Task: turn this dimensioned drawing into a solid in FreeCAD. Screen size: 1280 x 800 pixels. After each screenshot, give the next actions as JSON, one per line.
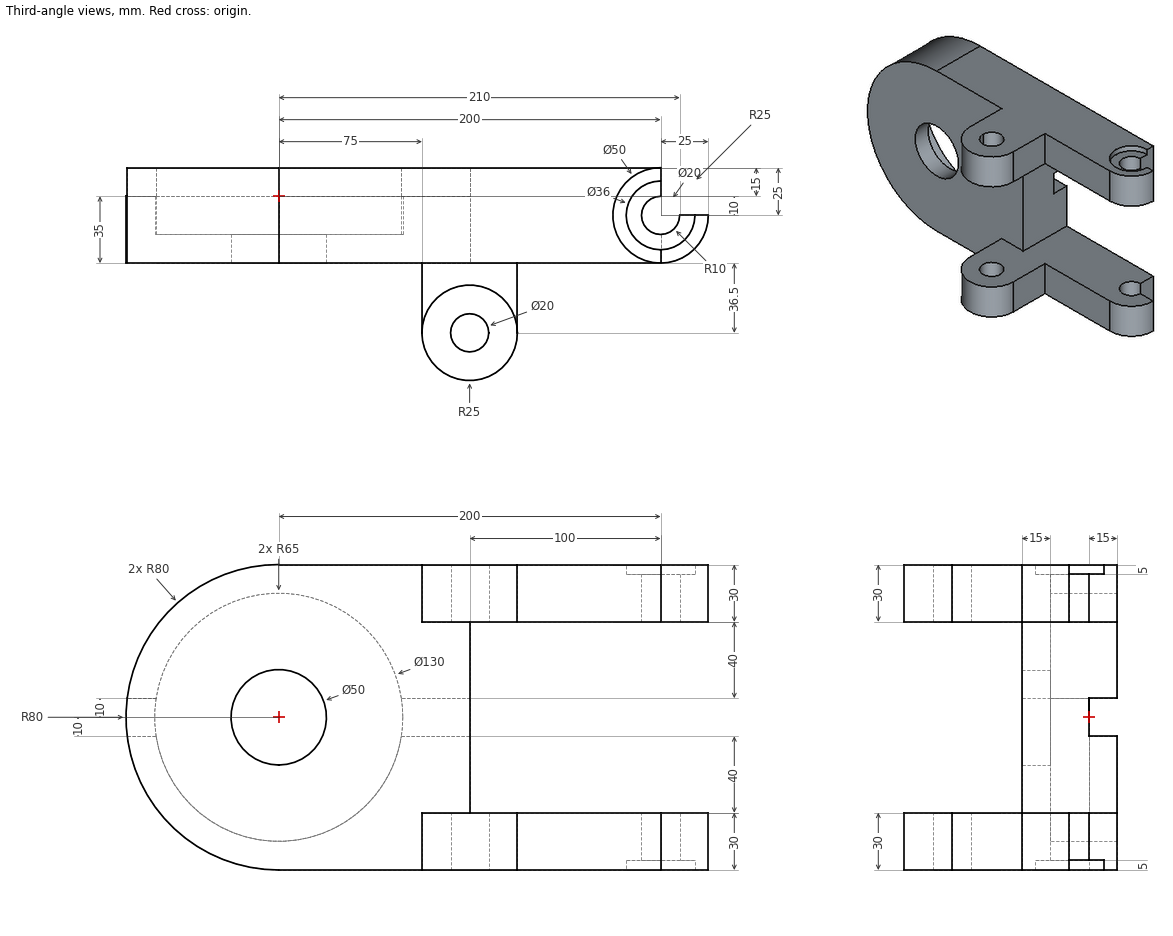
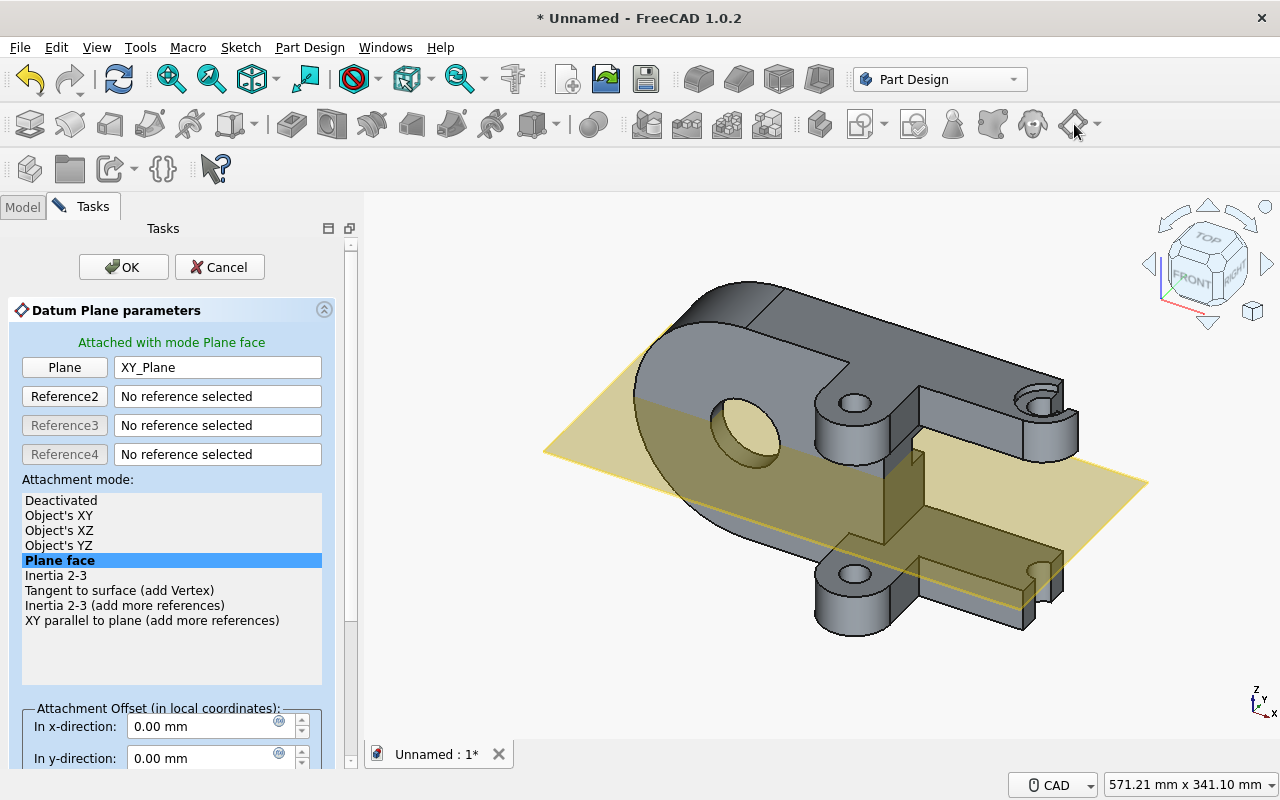
{"action": "scroll", "coordinate": [351, 503], "scroll_direction": "down", "scroll_amount": 2}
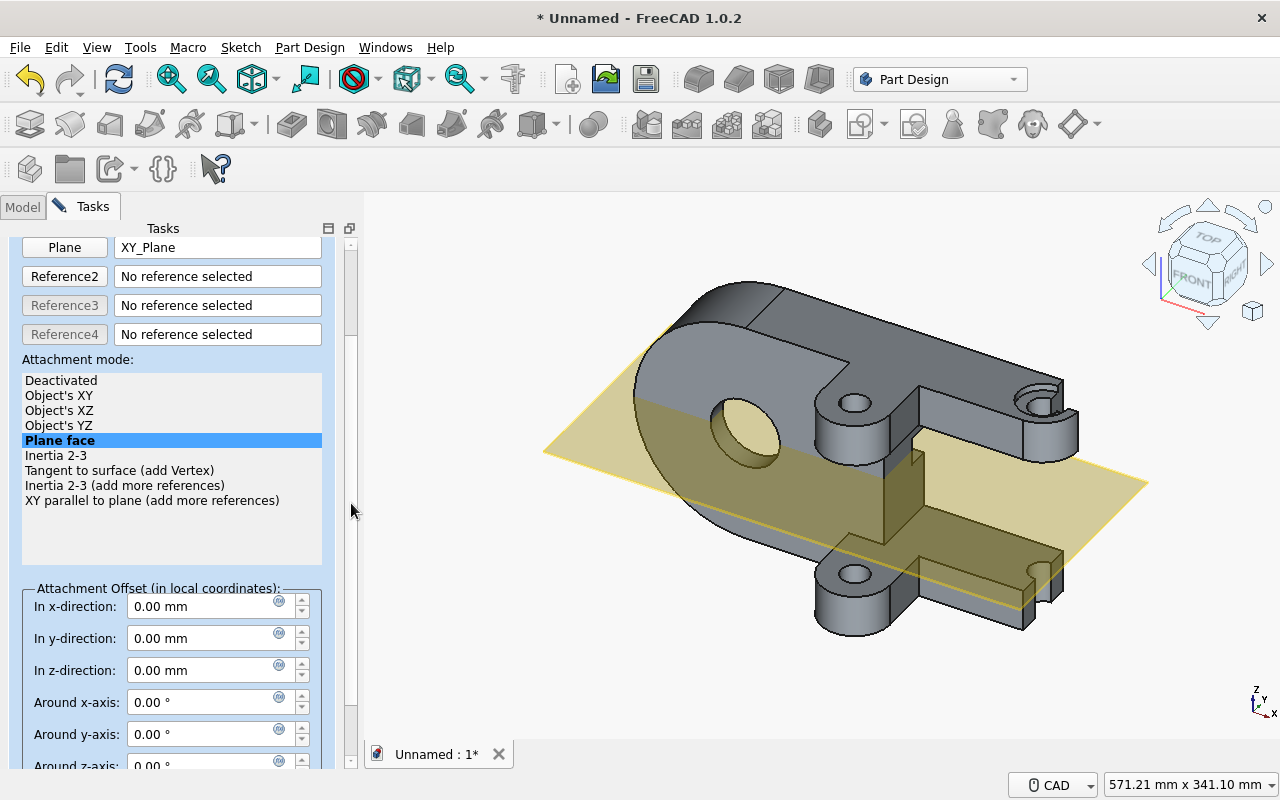
{"action": "triple_click", "coordinate": [210, 670]}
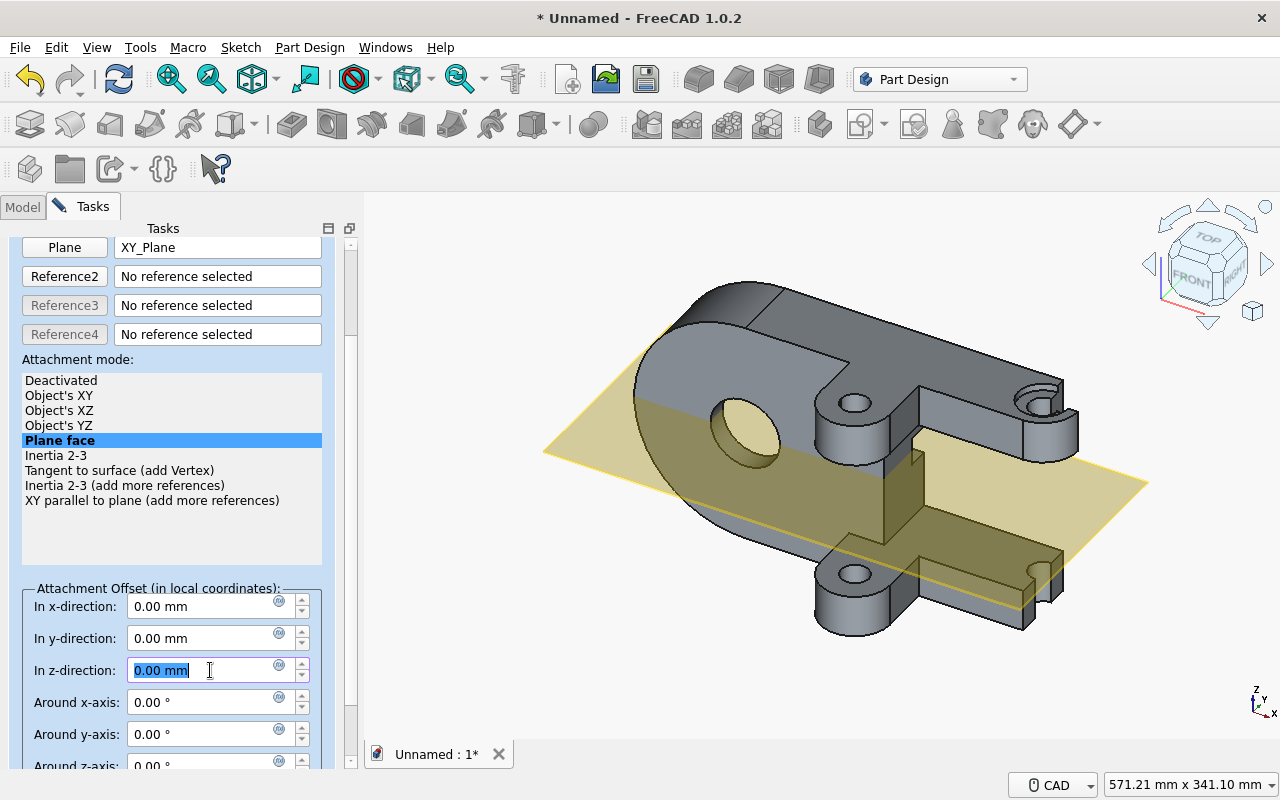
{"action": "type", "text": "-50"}
{"action": "key", "text": "Tab"}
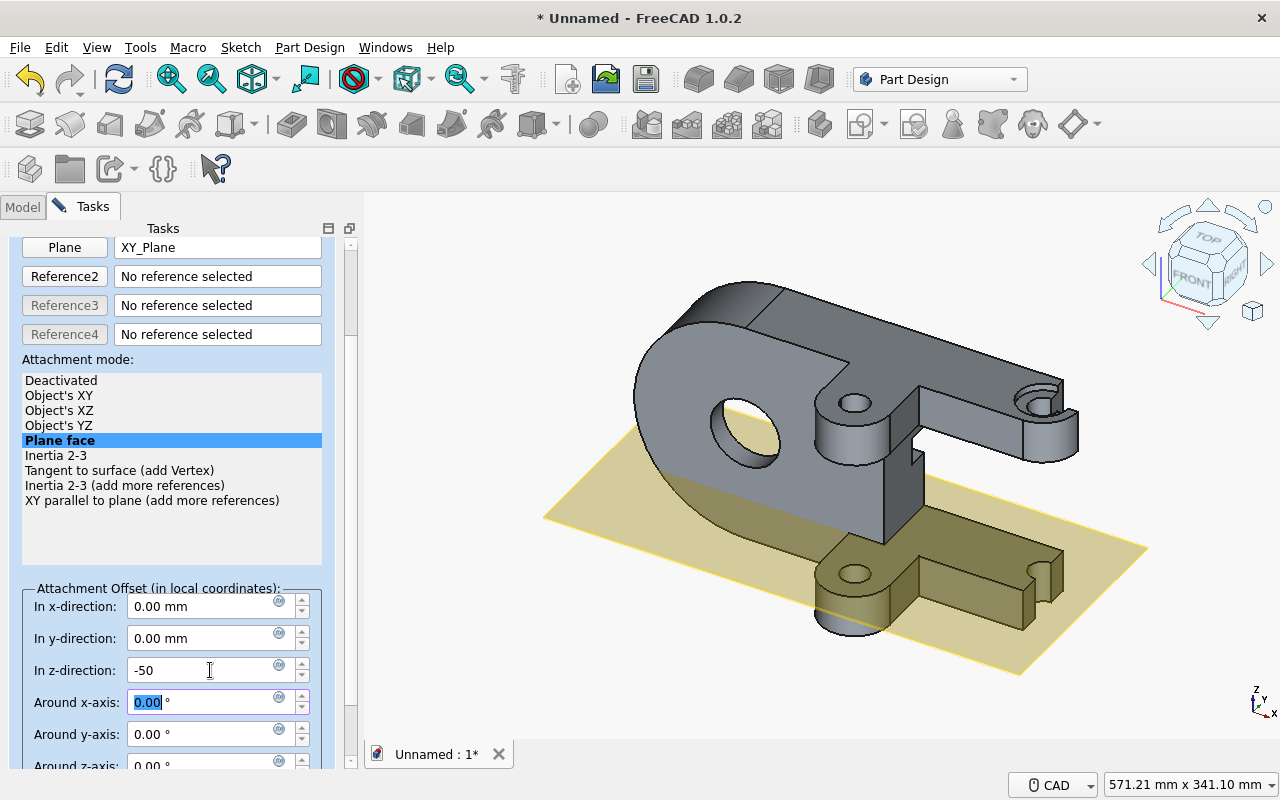
{"action": "scroll", "coordinate": [351, 503], "scroll_direction": "up", "scroll_amount": 3}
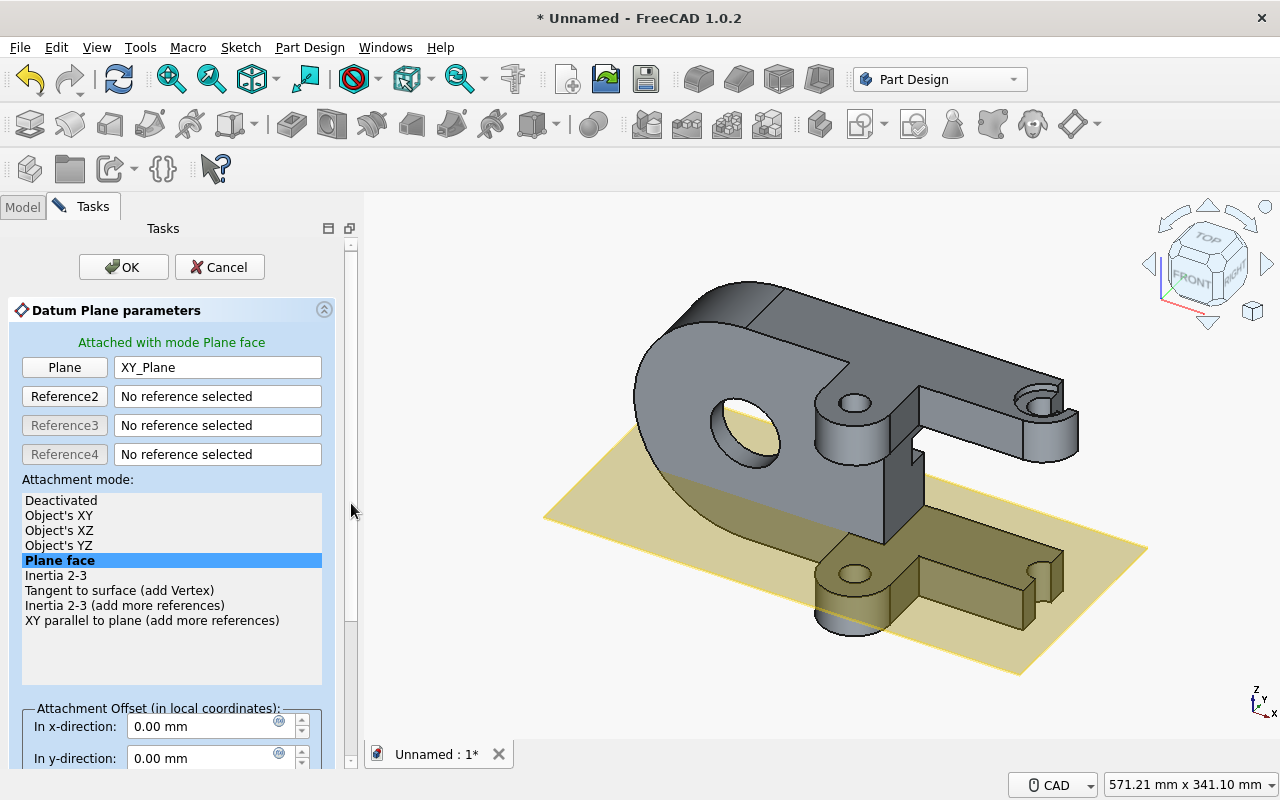
{"action": "left_click", "coordinate": [124, 267]}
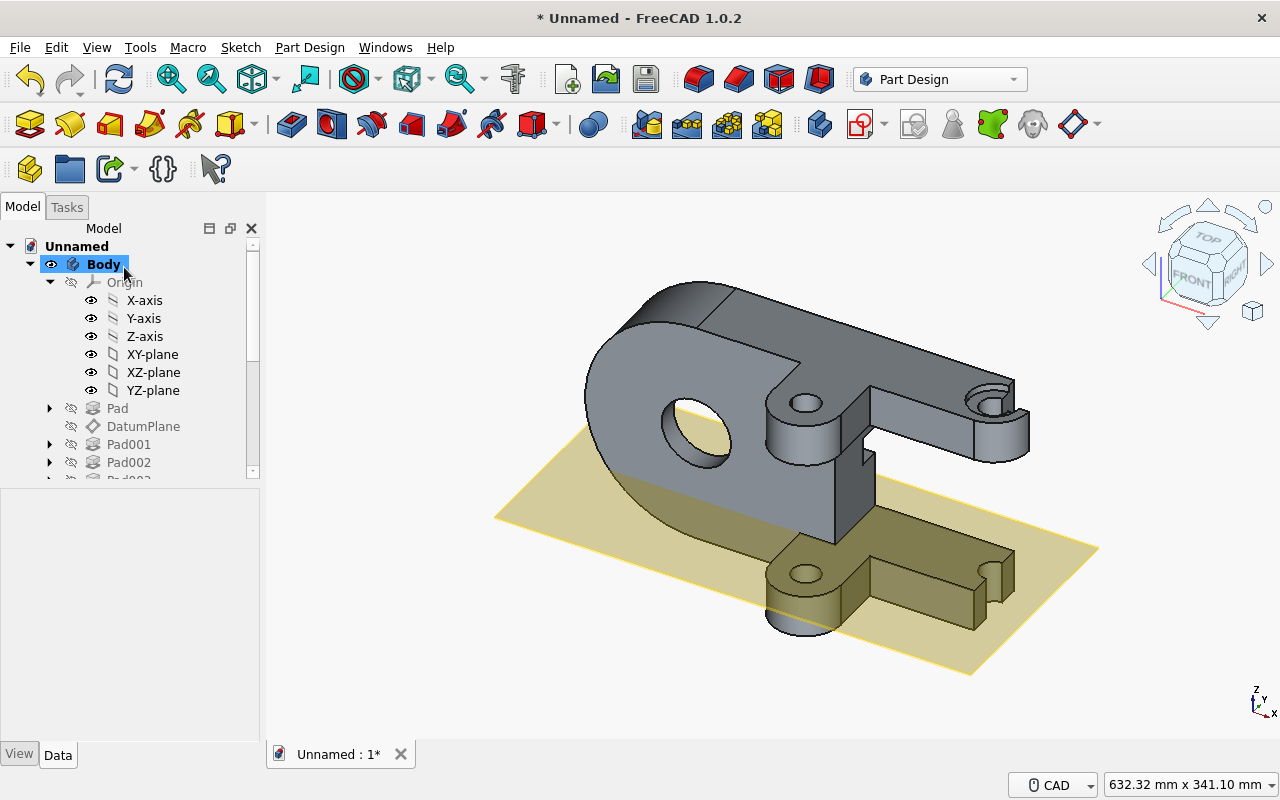
{"action": "scroll", "coordinate": [100, 350], "scroll_direction": "down", "scroll_amount": 3}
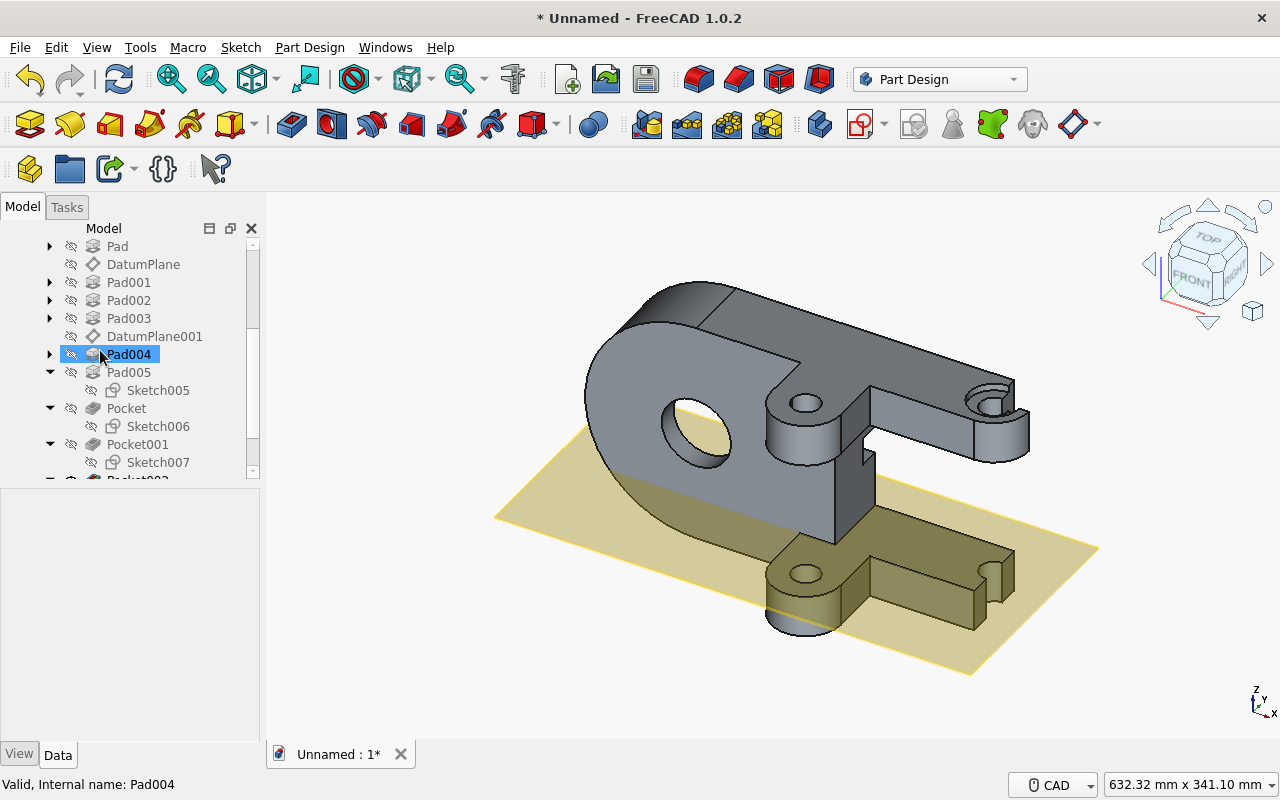
{"action": "scroll", "coordinate": [140, 350], "scroll_direction": "up", "scroll_amount": 15}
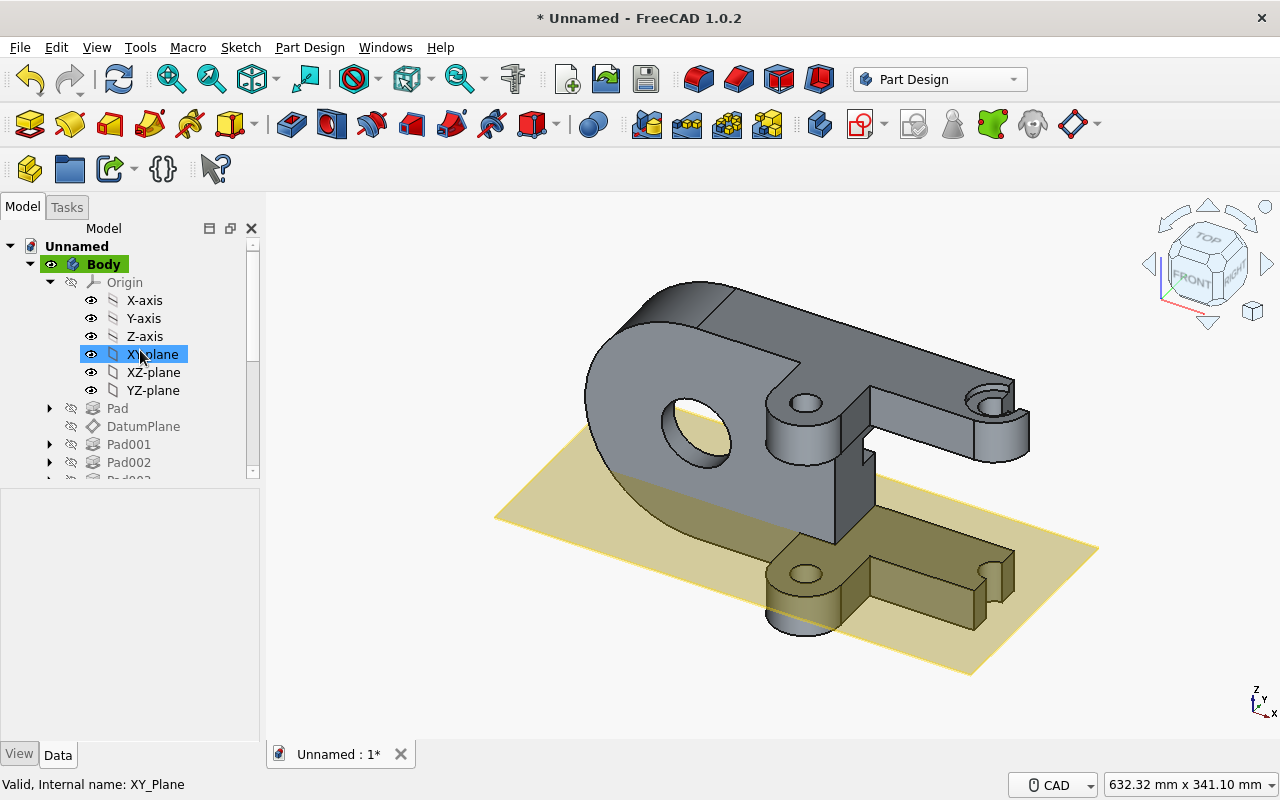
{"action": "scroll", "coordinate": [100, 350], "scroll_direction": "down", "scroll_amount": 6}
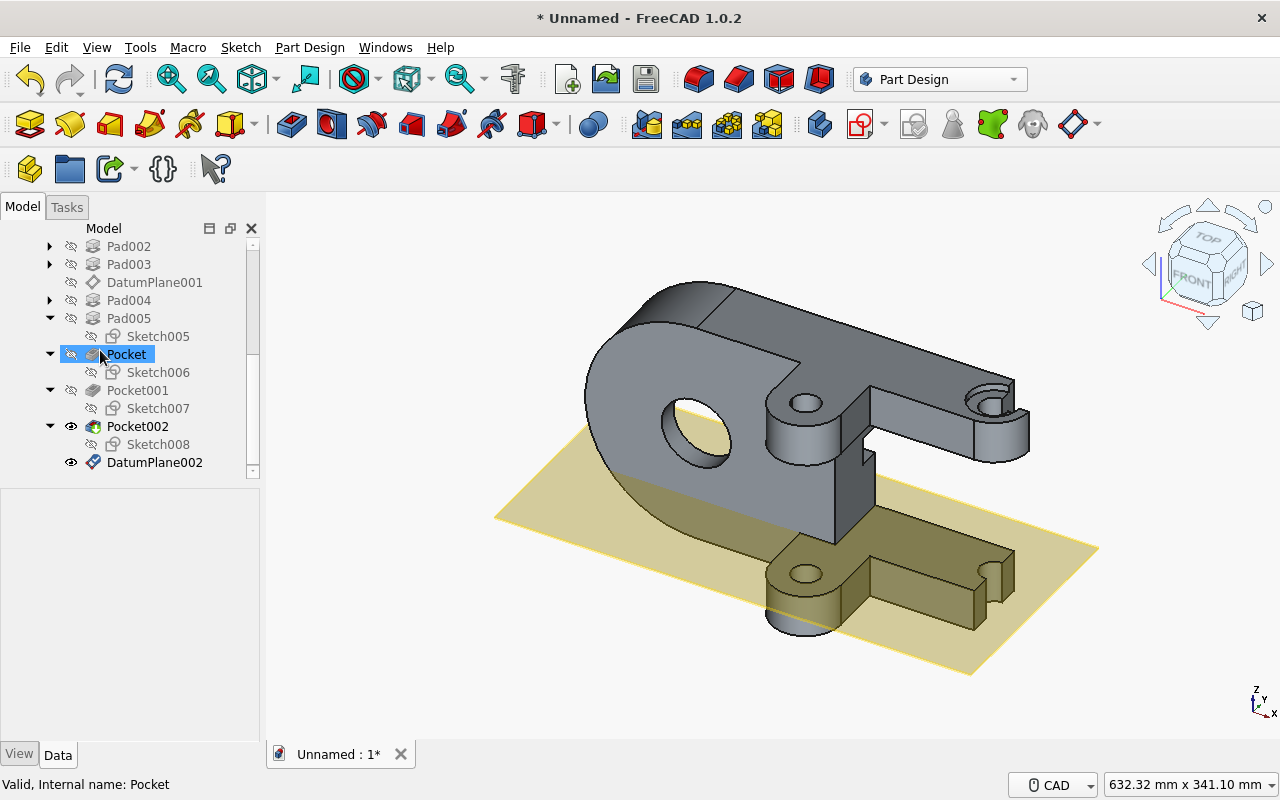
{"action": "left_click", "coordinate": [116, 462]}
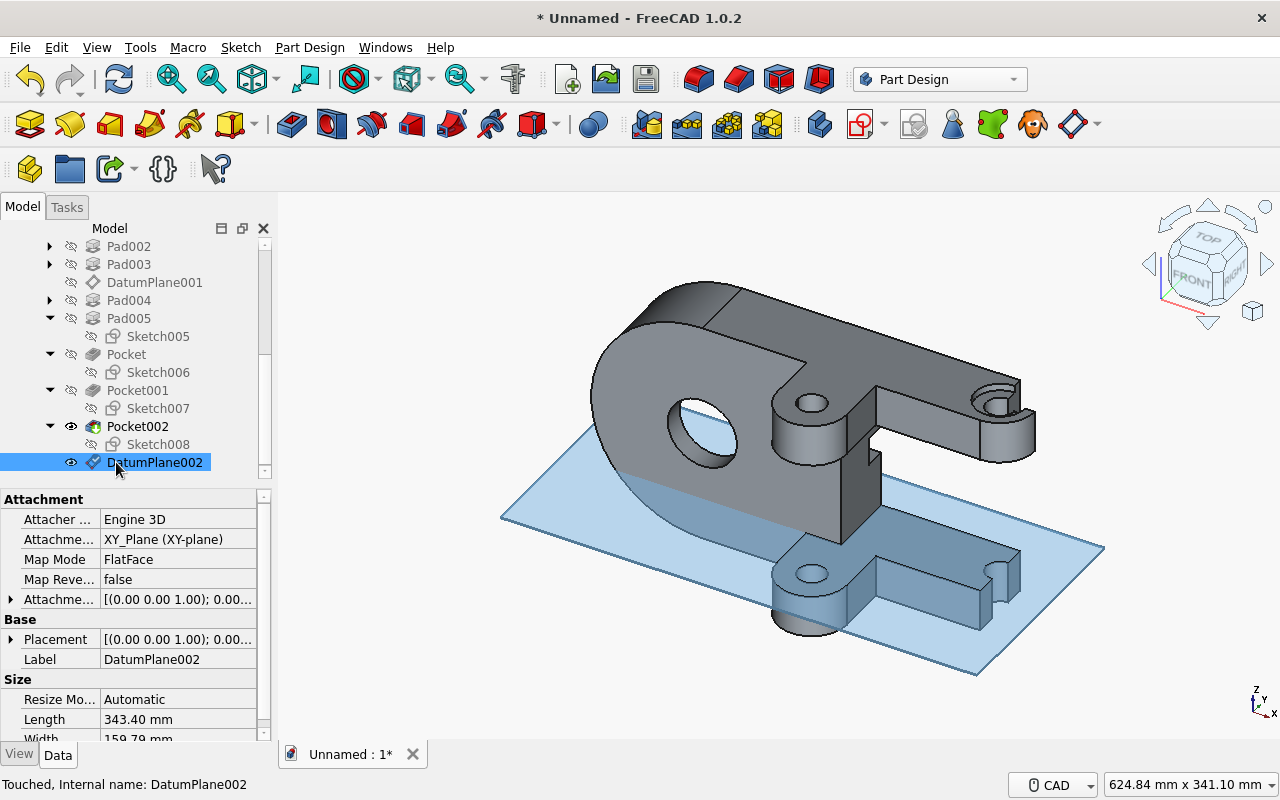
{"action": "left_click", "coordinate": [860, 124]}